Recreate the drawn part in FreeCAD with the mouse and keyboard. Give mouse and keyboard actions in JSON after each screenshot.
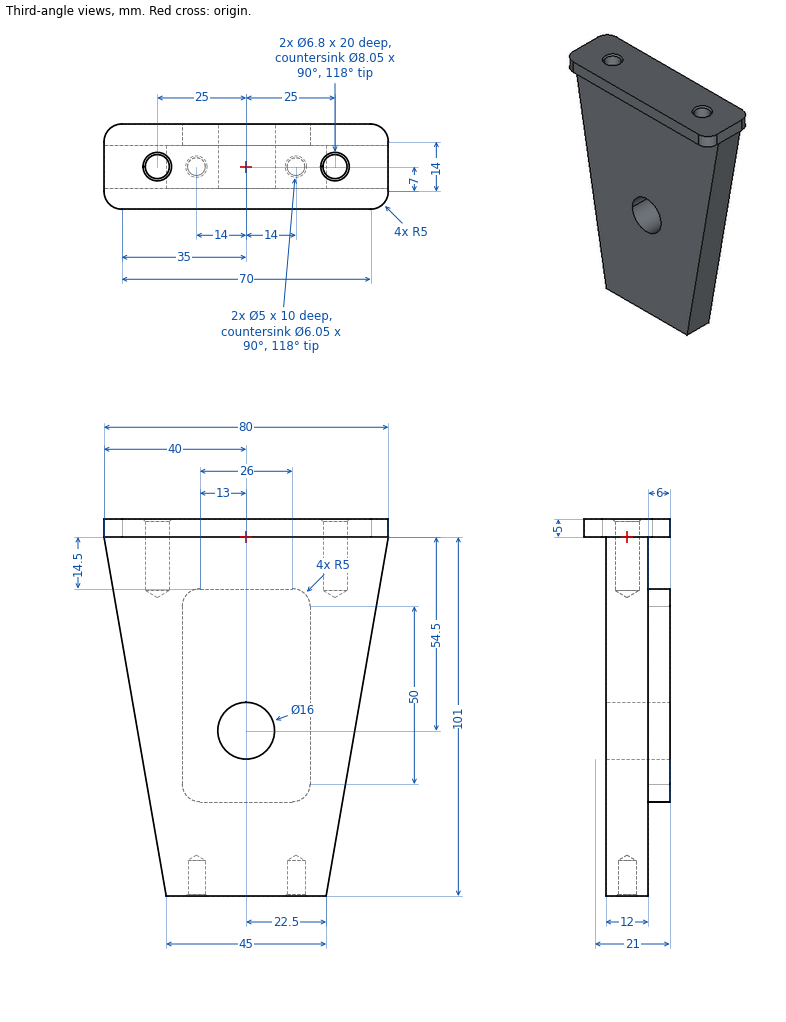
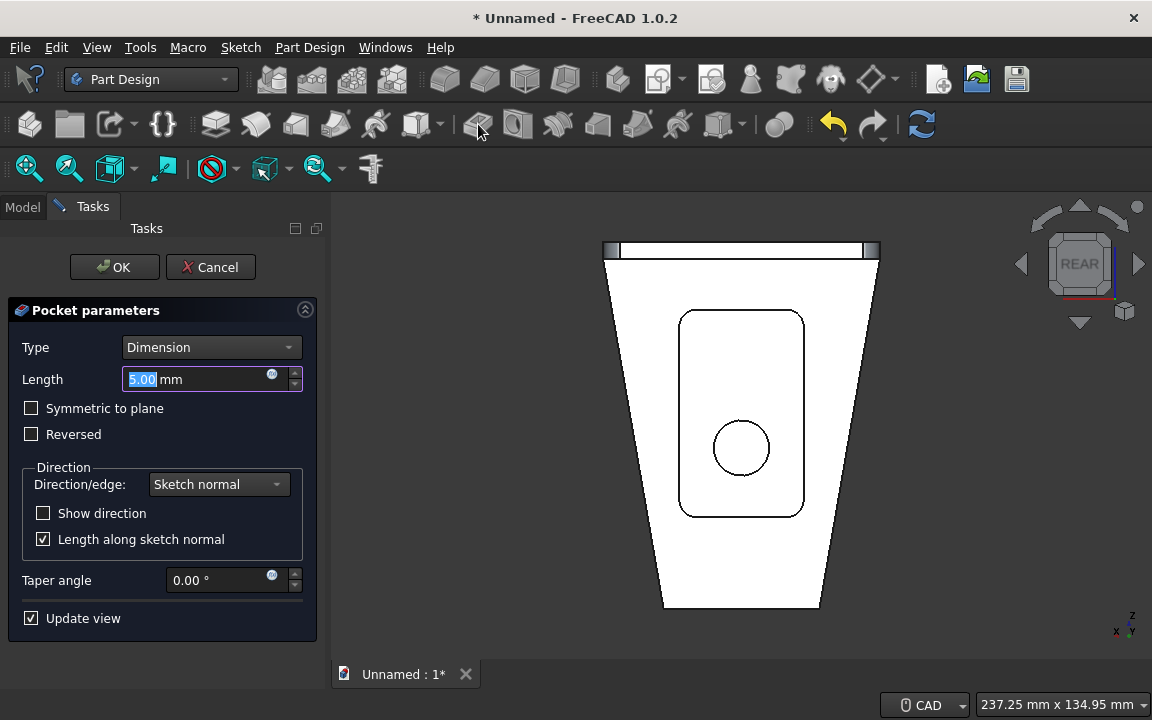
{"action": "type", "text": "21"}
{"action": "key", "text": "Tab"}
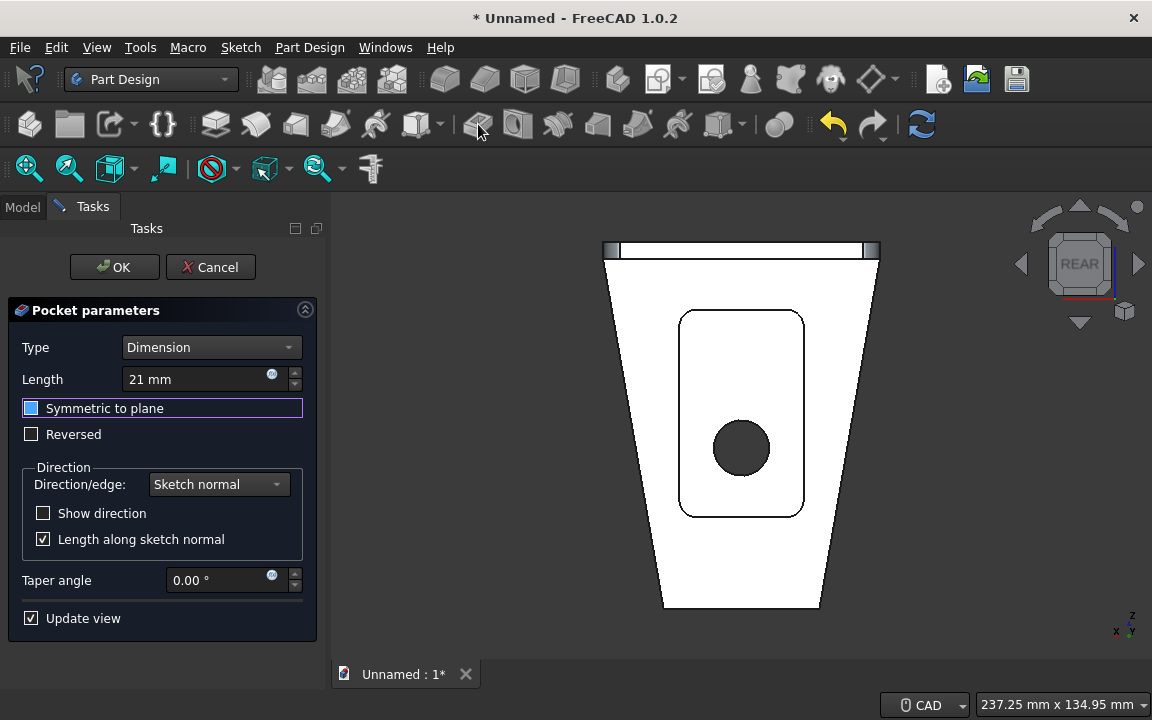
{"action": "left_click", "coordinate": [115, 267]}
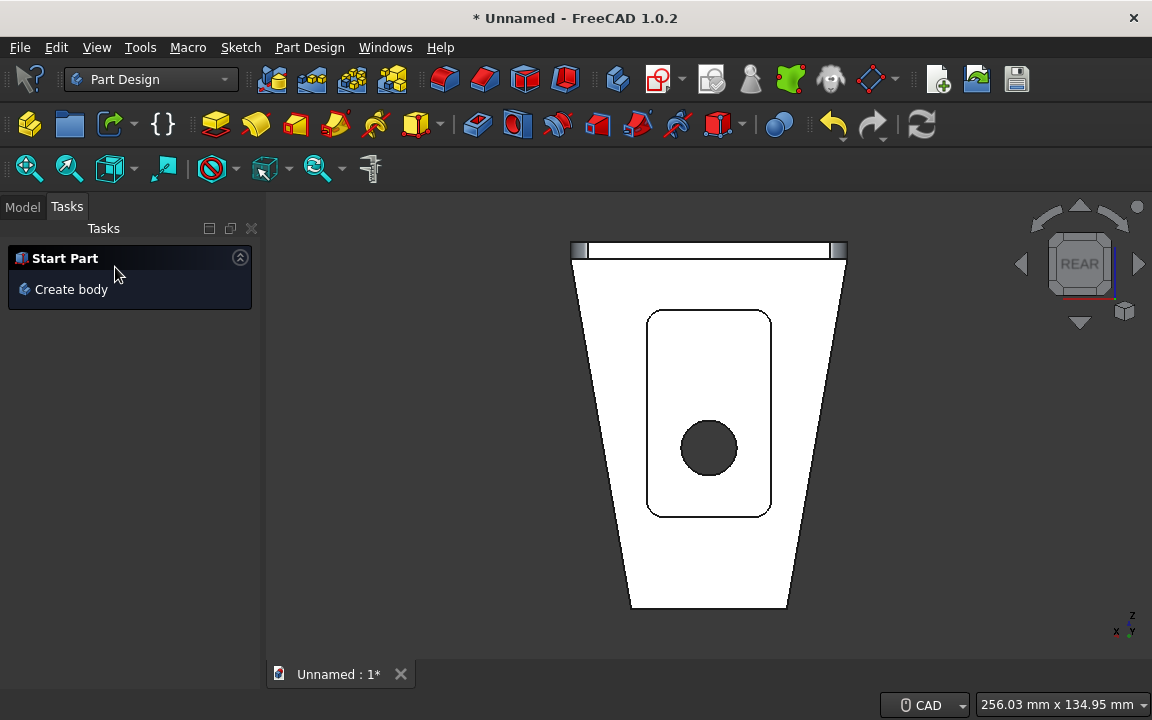
{"action": "key", "text": "0"}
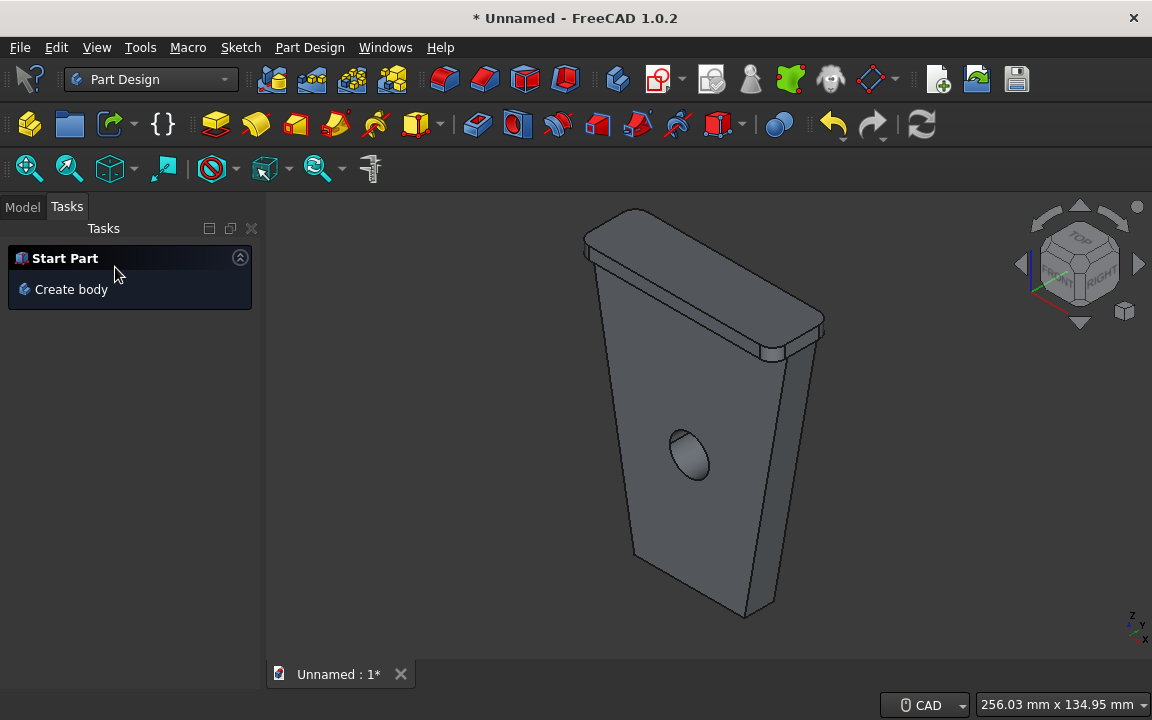
{"action": "left_click", "coordinate": [760, 310]}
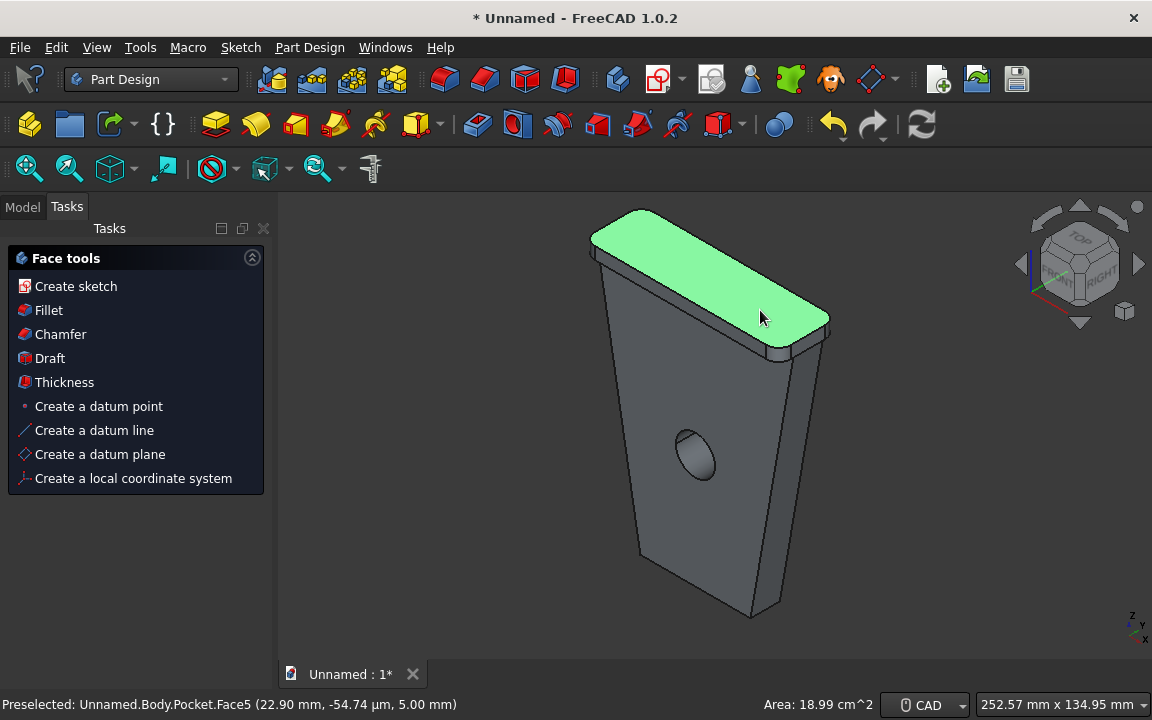
{"action": "left_click", "coordinate": [658, 80]}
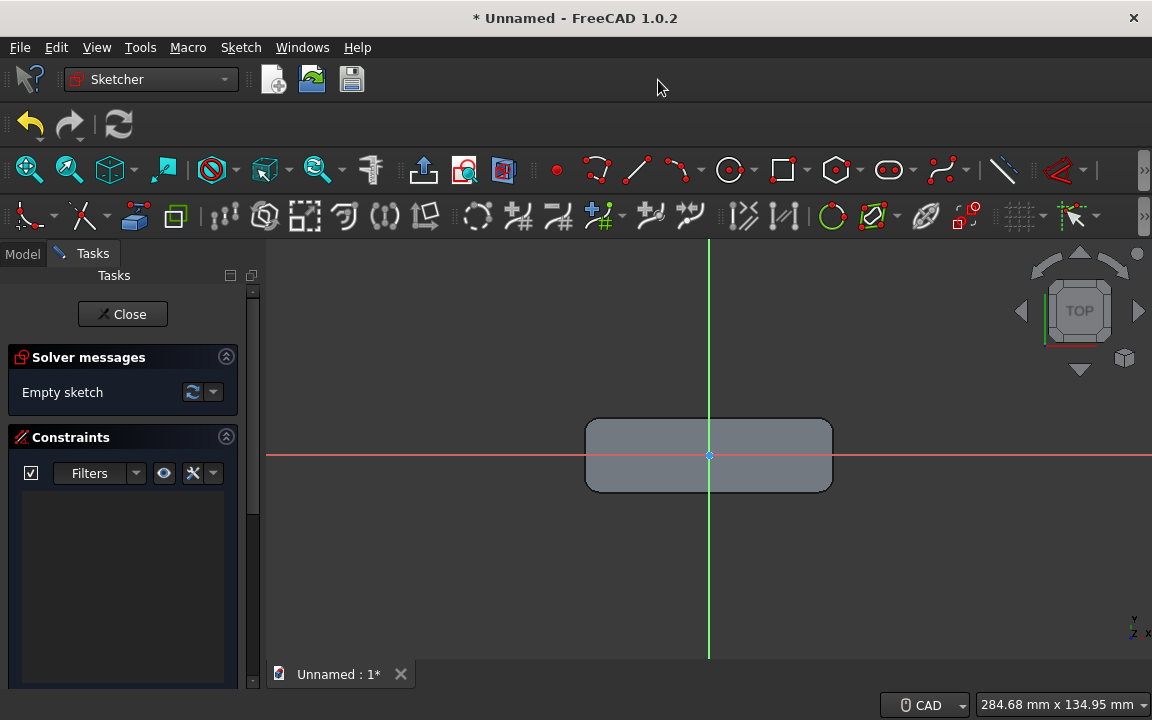
{"action": "scroll", "coordinate": [749, 459], "scroll_direction": "up", "scroll_amount": 5}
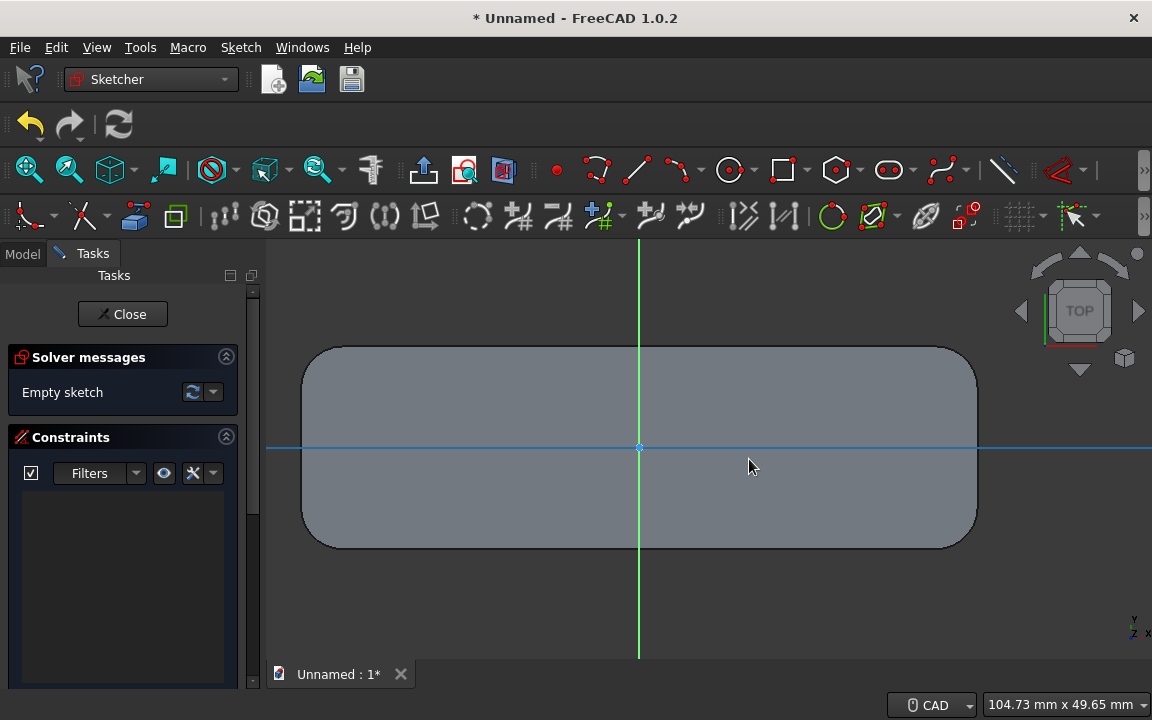
{"action": "left_click", "coordinate": [730, 170]}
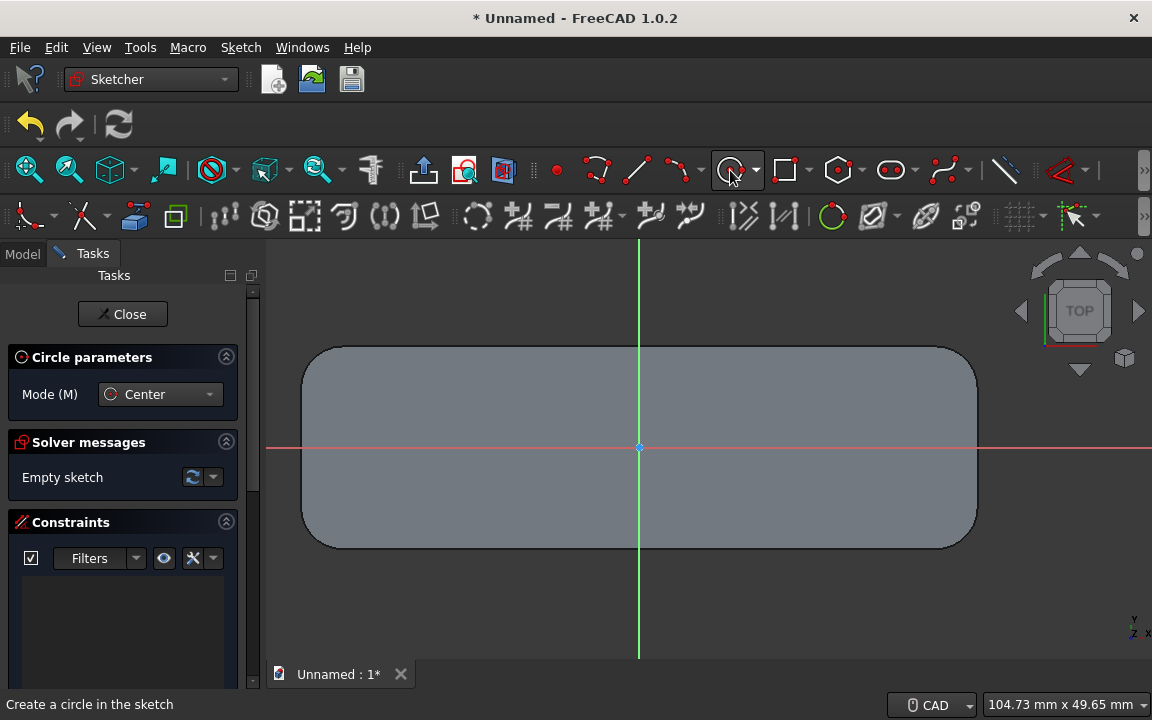
{"action": "left_click", "coordinate": [851, 448]}
{"action": "mouse_move", "coordinate": [871, 427]}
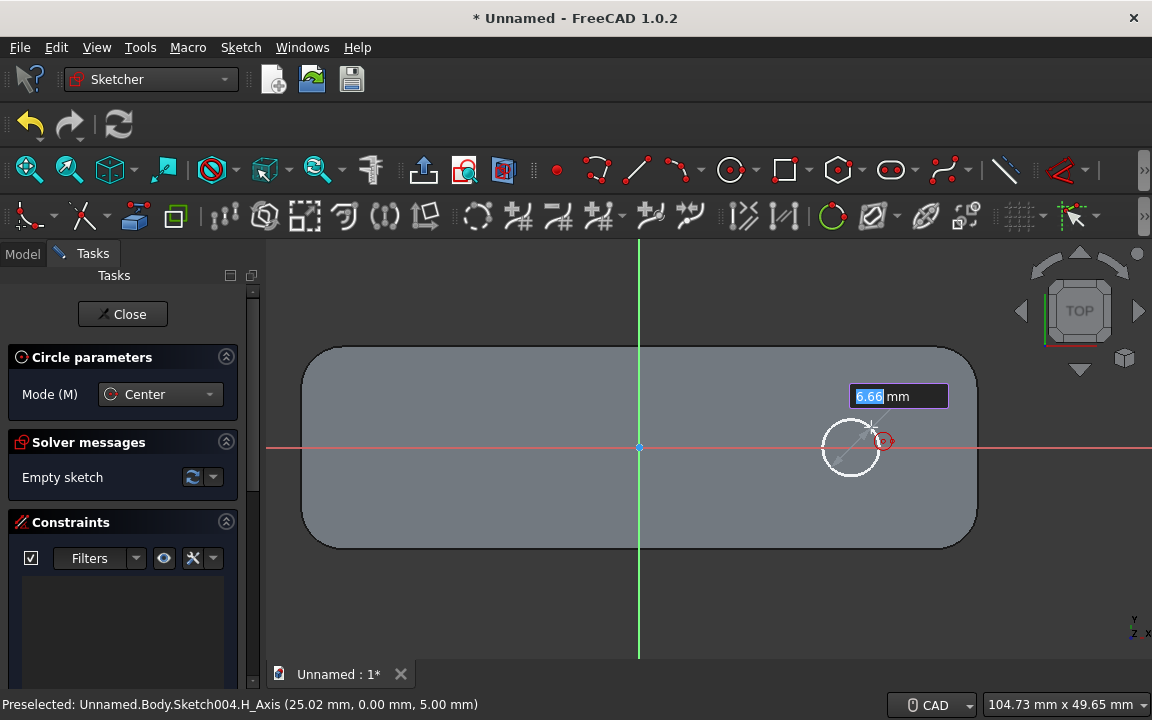
{"action": "type", "text": "6.8"}
{"action": "key", "text": "Return"}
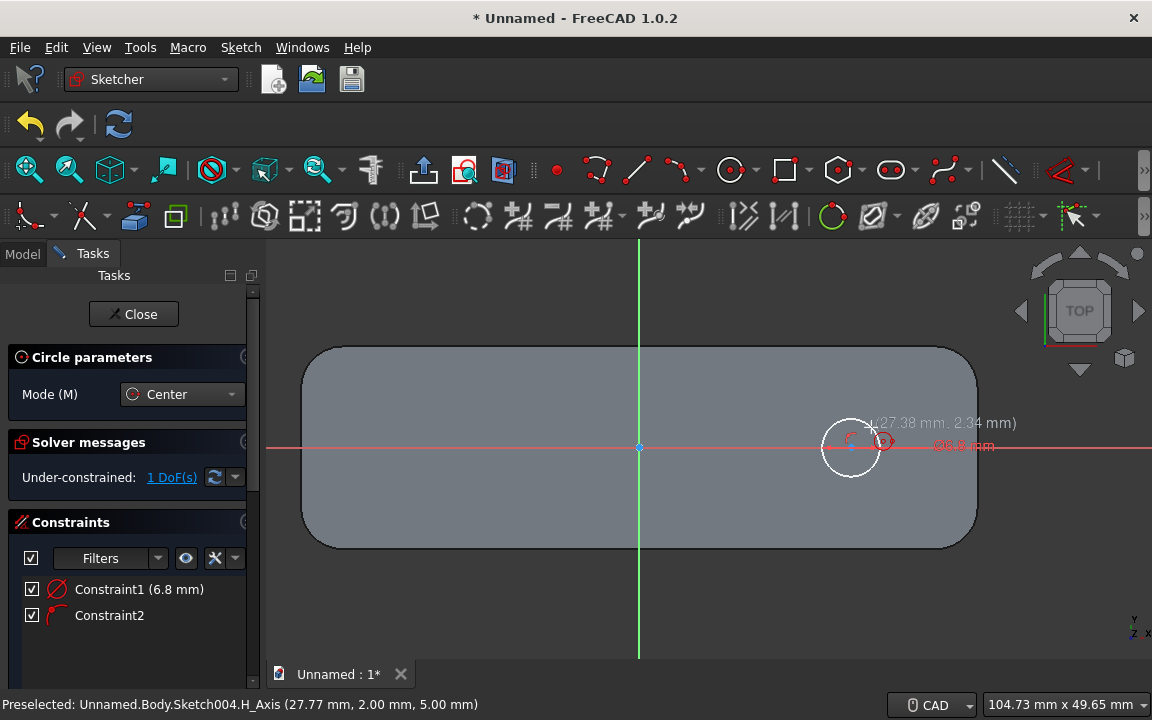
{"action": "left_click", "coordinate": [428, 448]}
{"action": "mouse_move", "coordinate": [448, 427]}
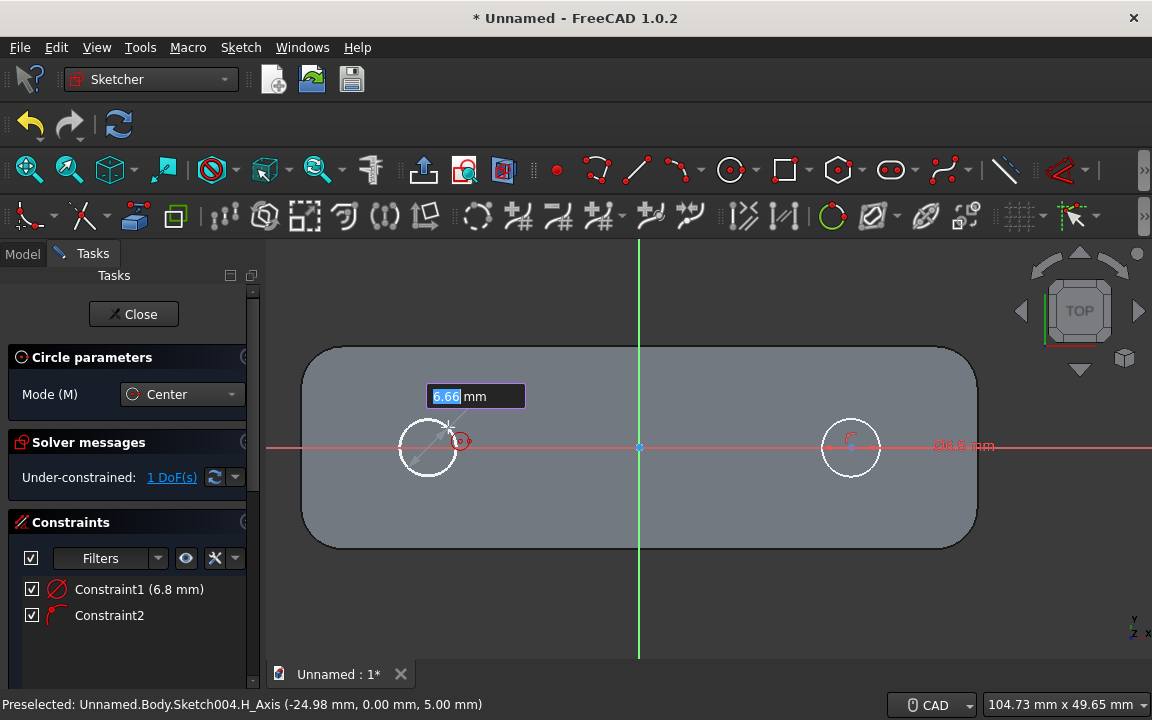
{"action": "type", "text": "6.8"}
{"action": "key", "text": "Return"}
{"action": "key", "text": "Escape"}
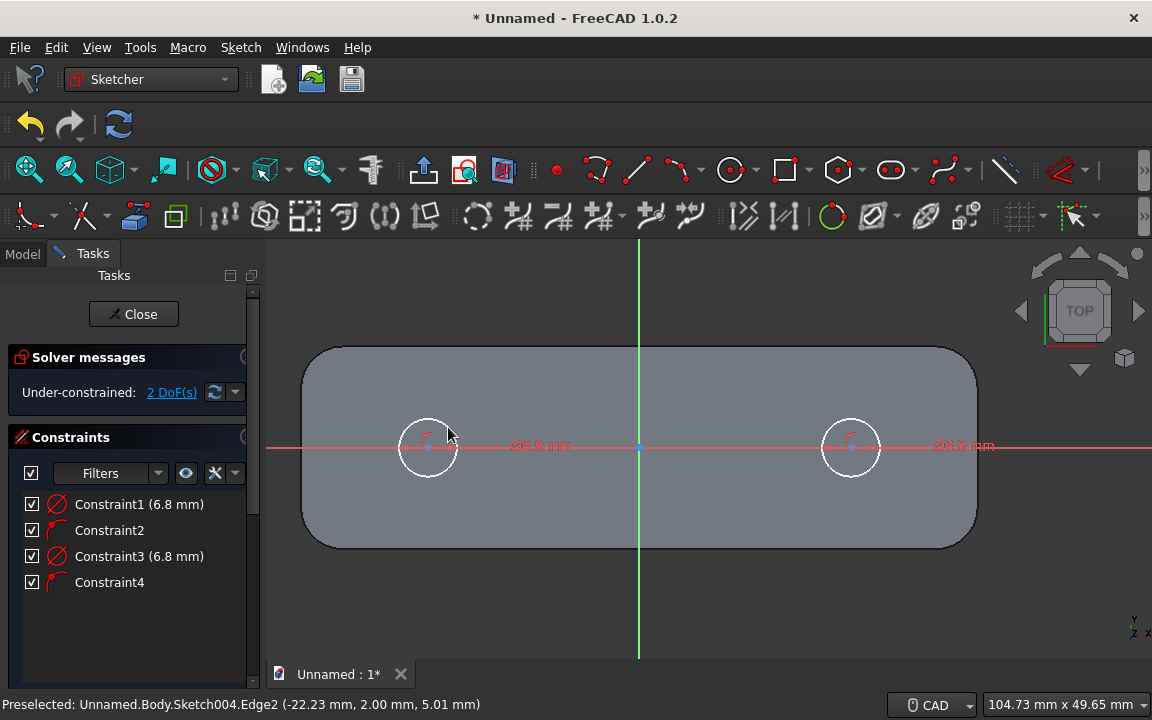
{"action": "left_click", "coordinate": [1060, 170]}